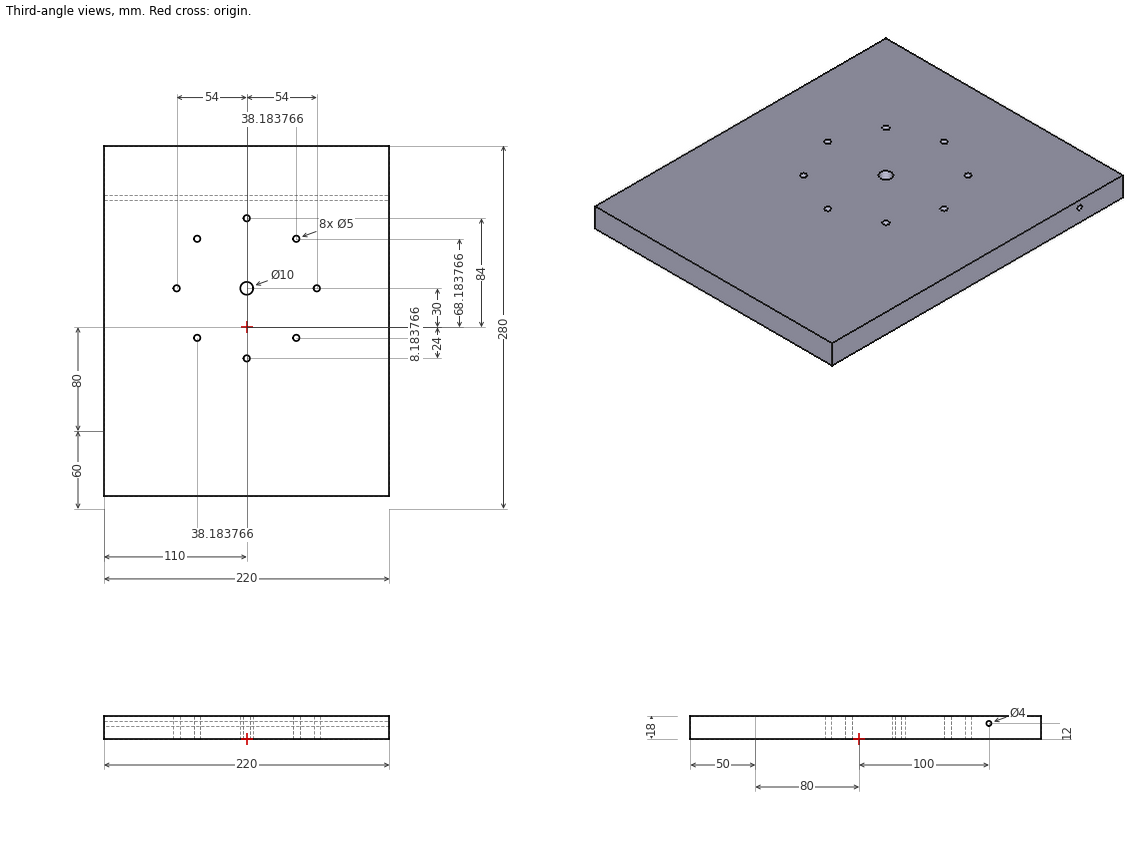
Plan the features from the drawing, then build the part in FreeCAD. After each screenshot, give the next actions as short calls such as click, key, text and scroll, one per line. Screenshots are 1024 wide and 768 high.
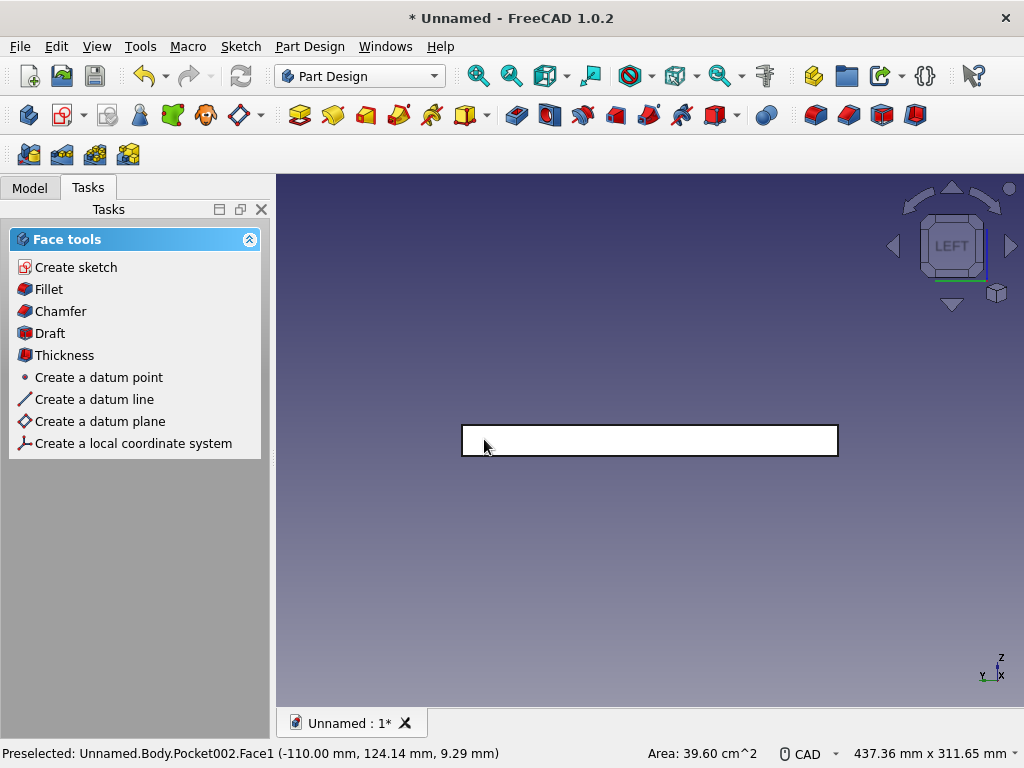
click(62, 116)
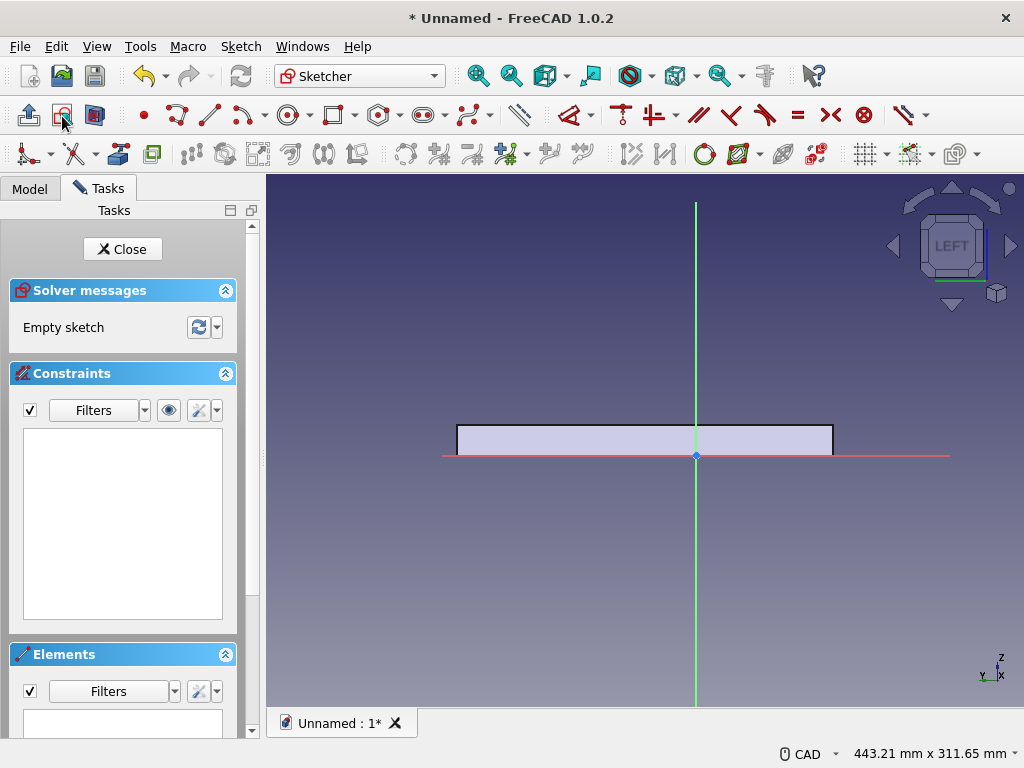
scroll(576, 440, down, 5)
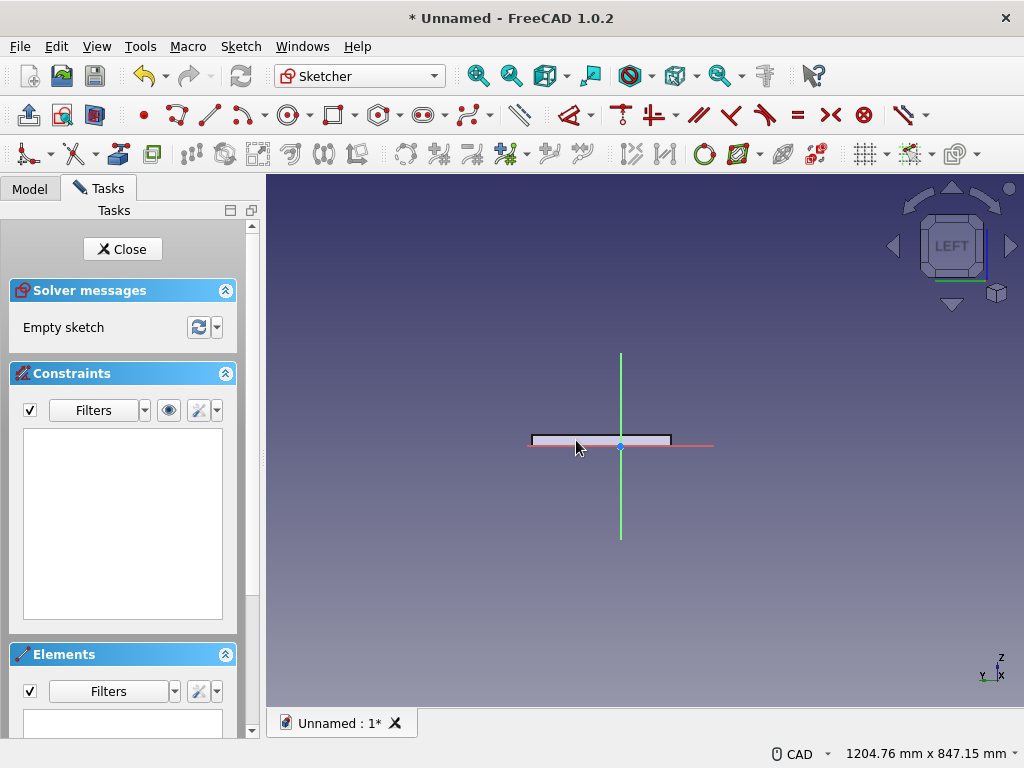
scroll(695, 440, up, 13)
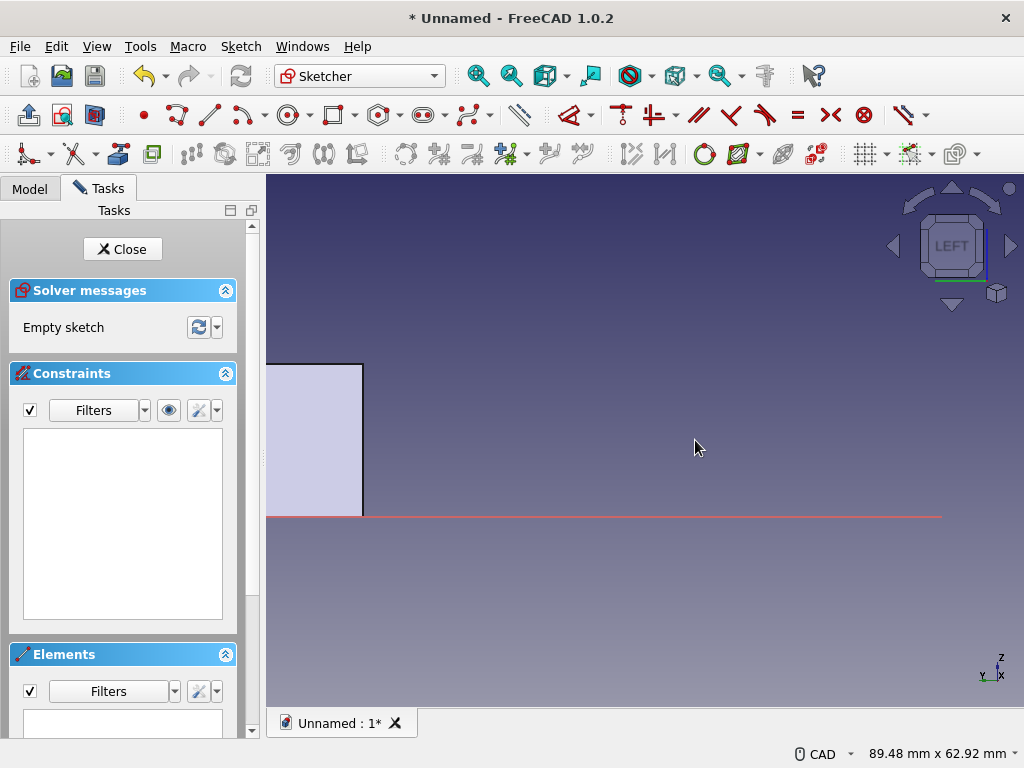
key(g)
key(r)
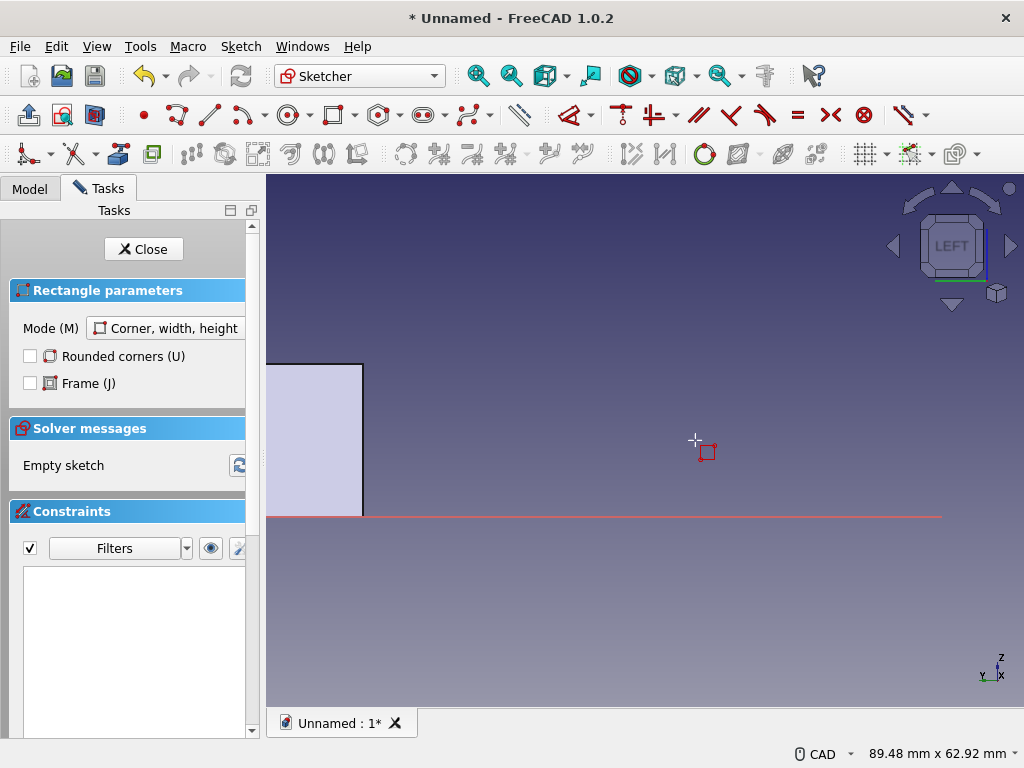
click(363, 364)
click(786, 517)
key(Escape)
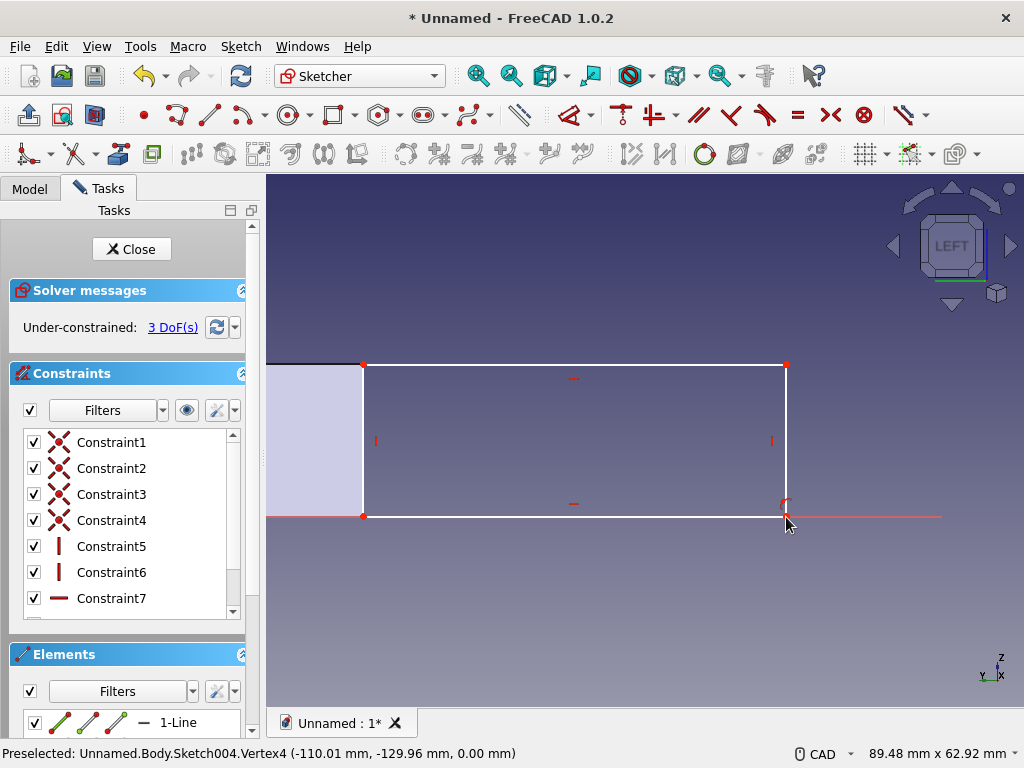
key(d)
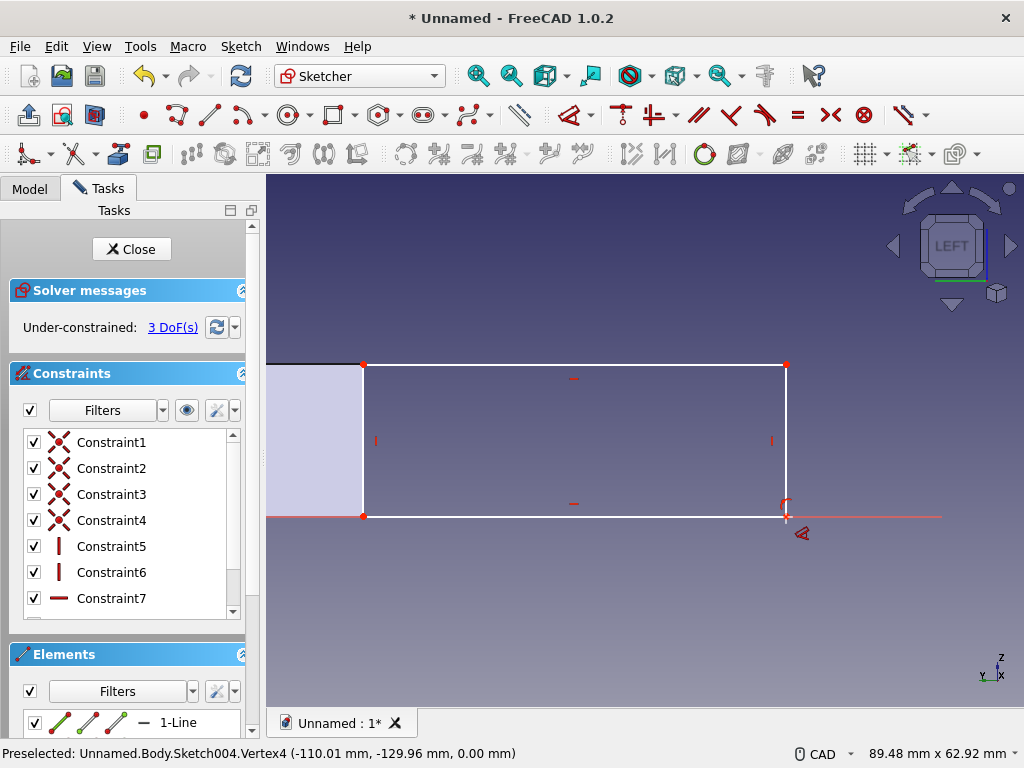
click(363, 411)
click(329, 441)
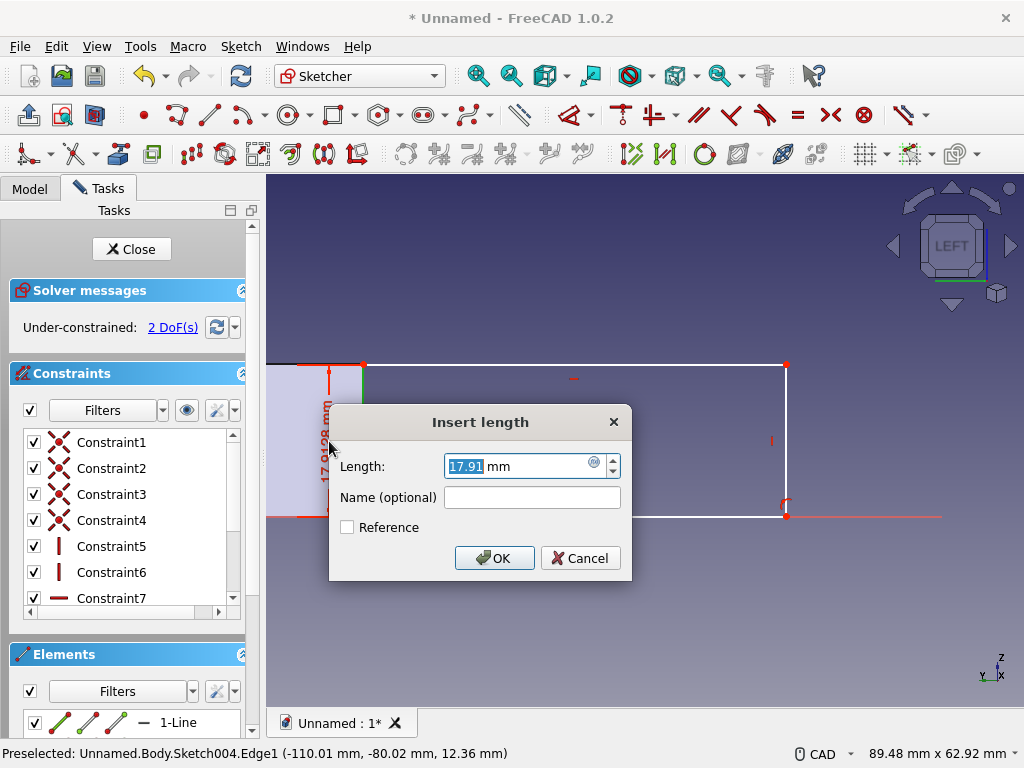
text(18)
key(Return)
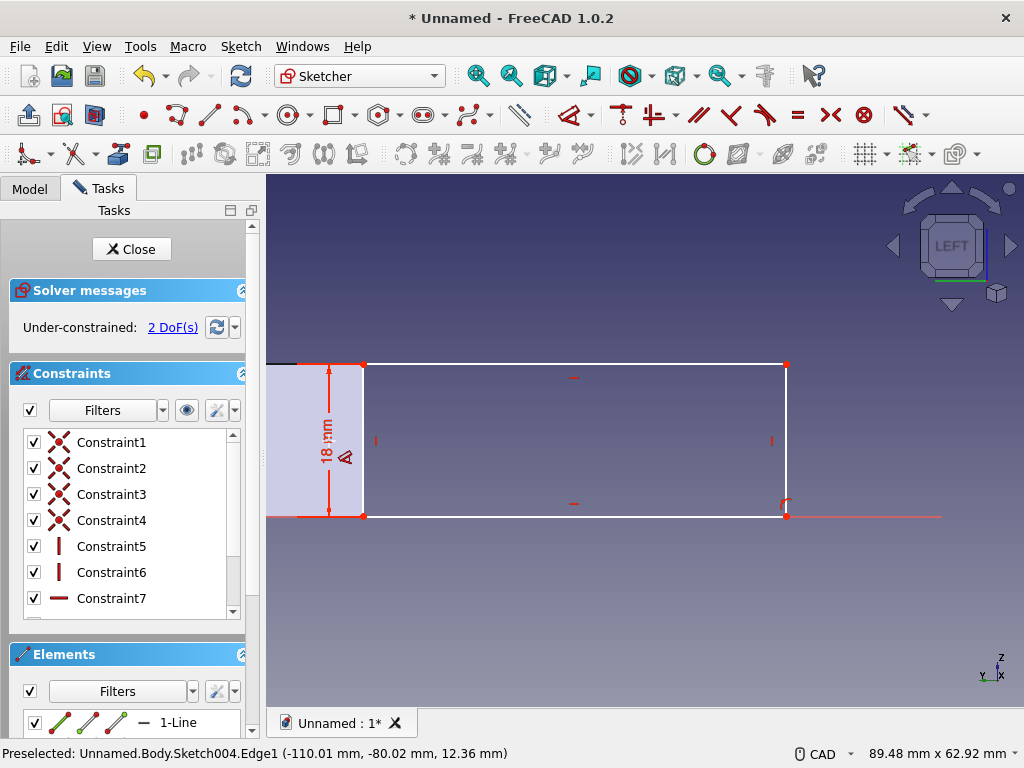
click(490, 517)
click(575, 551)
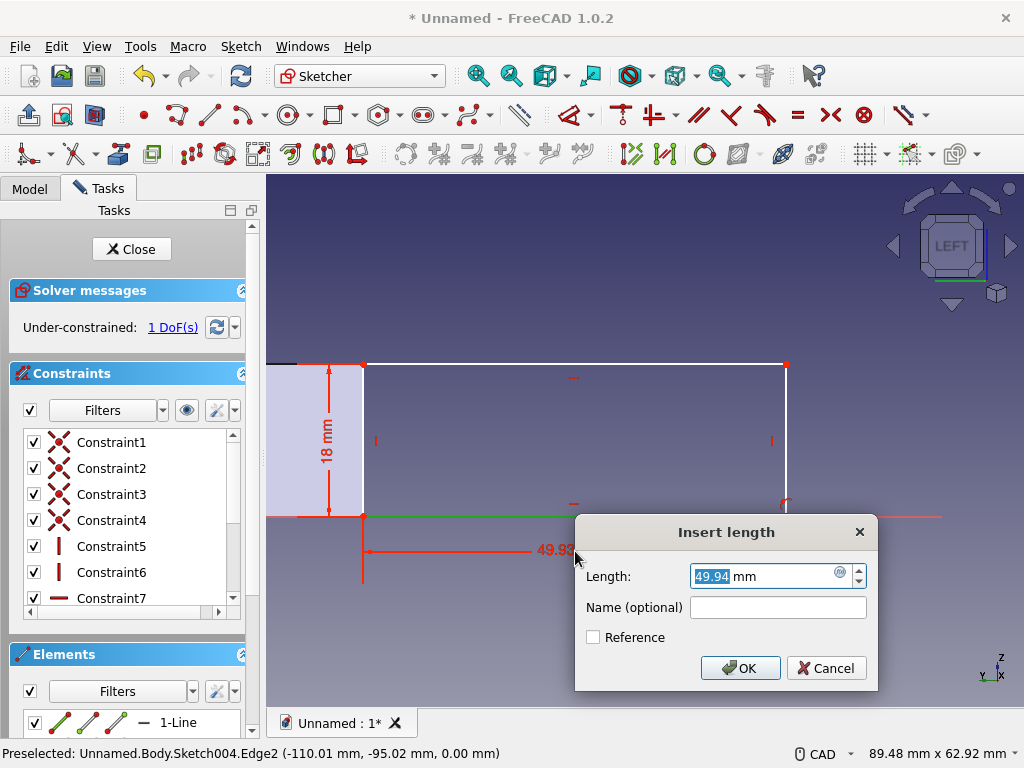
text(50)
key(Return)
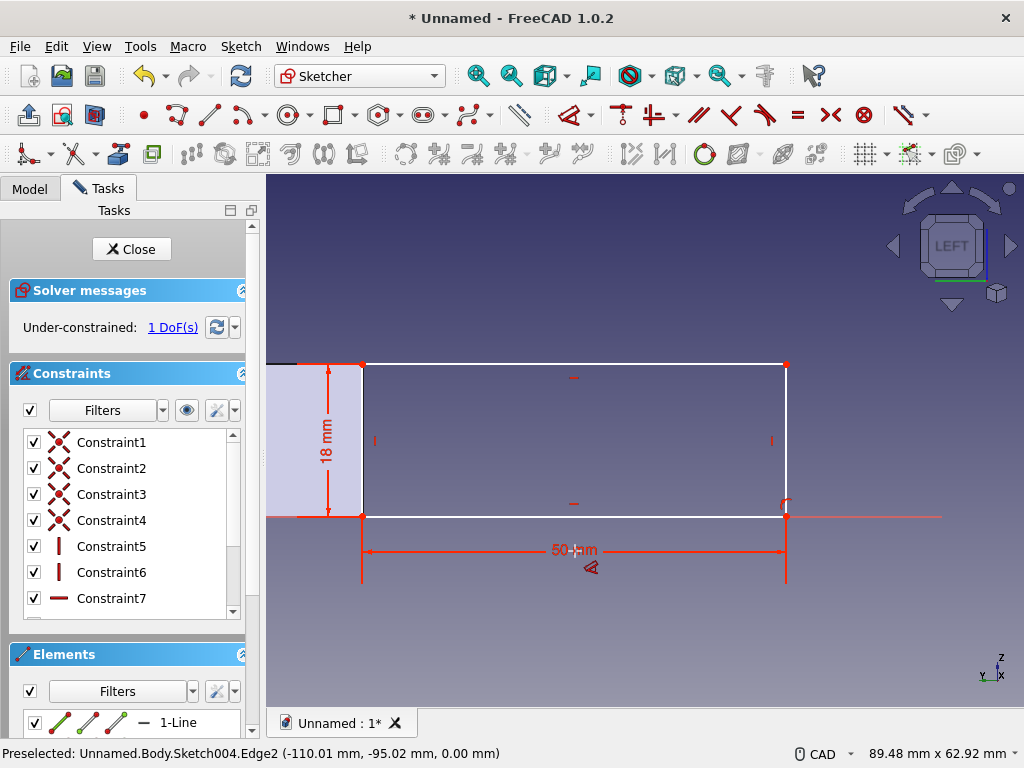
click(362, 364)
click(328, 551)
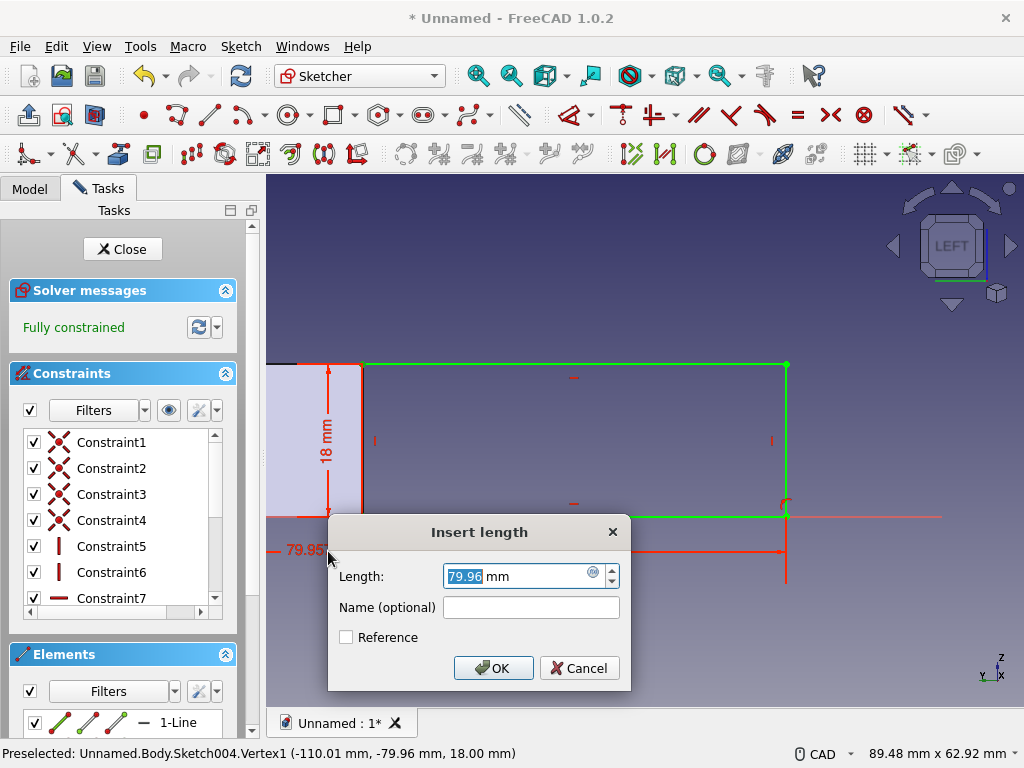
text(80)
key(Return)
key(Escape)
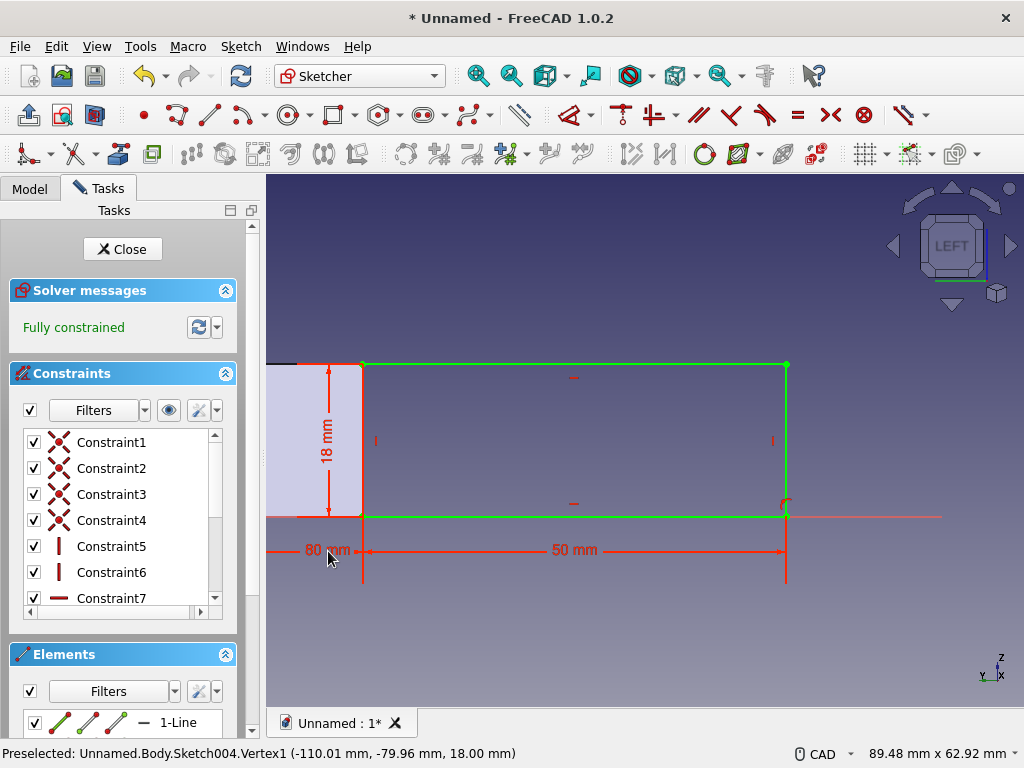
click(123, 249)